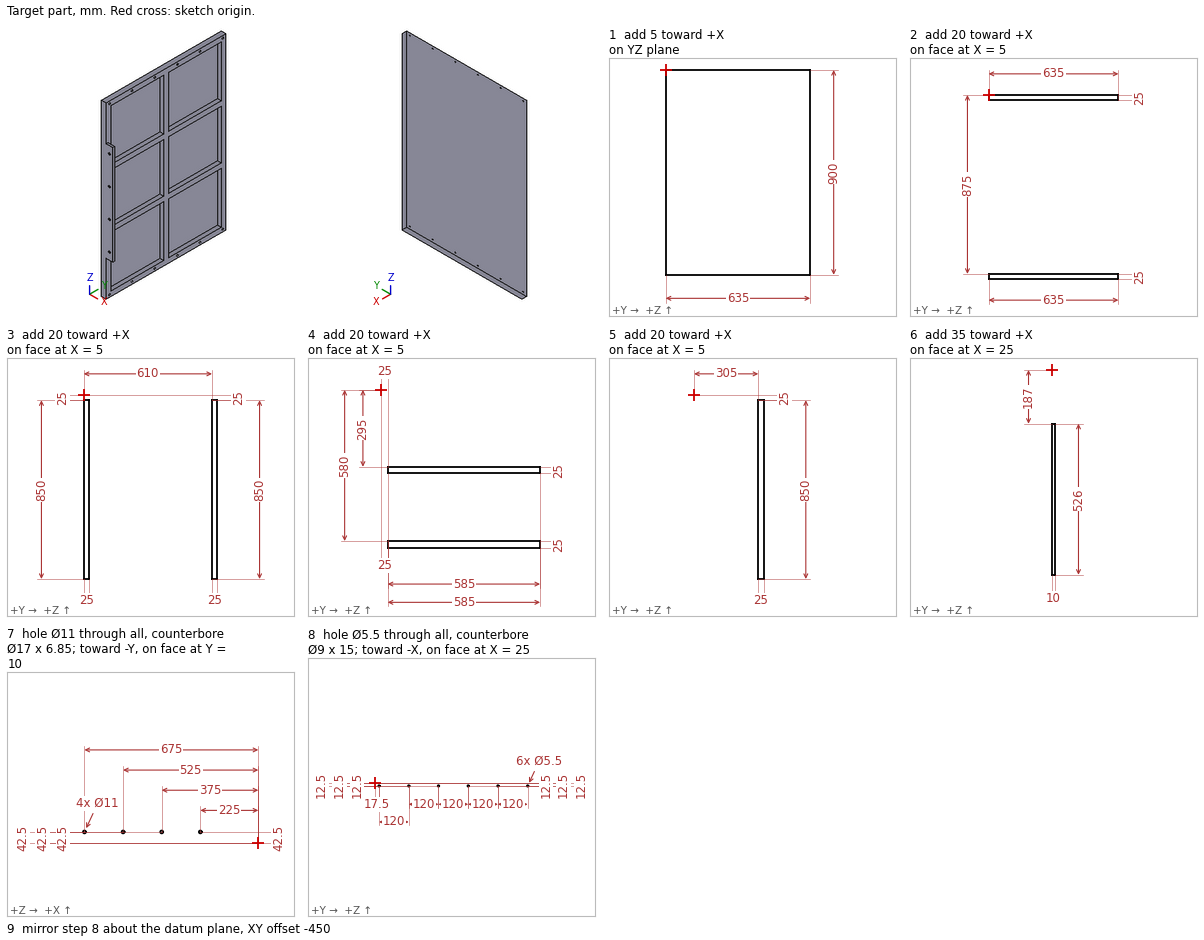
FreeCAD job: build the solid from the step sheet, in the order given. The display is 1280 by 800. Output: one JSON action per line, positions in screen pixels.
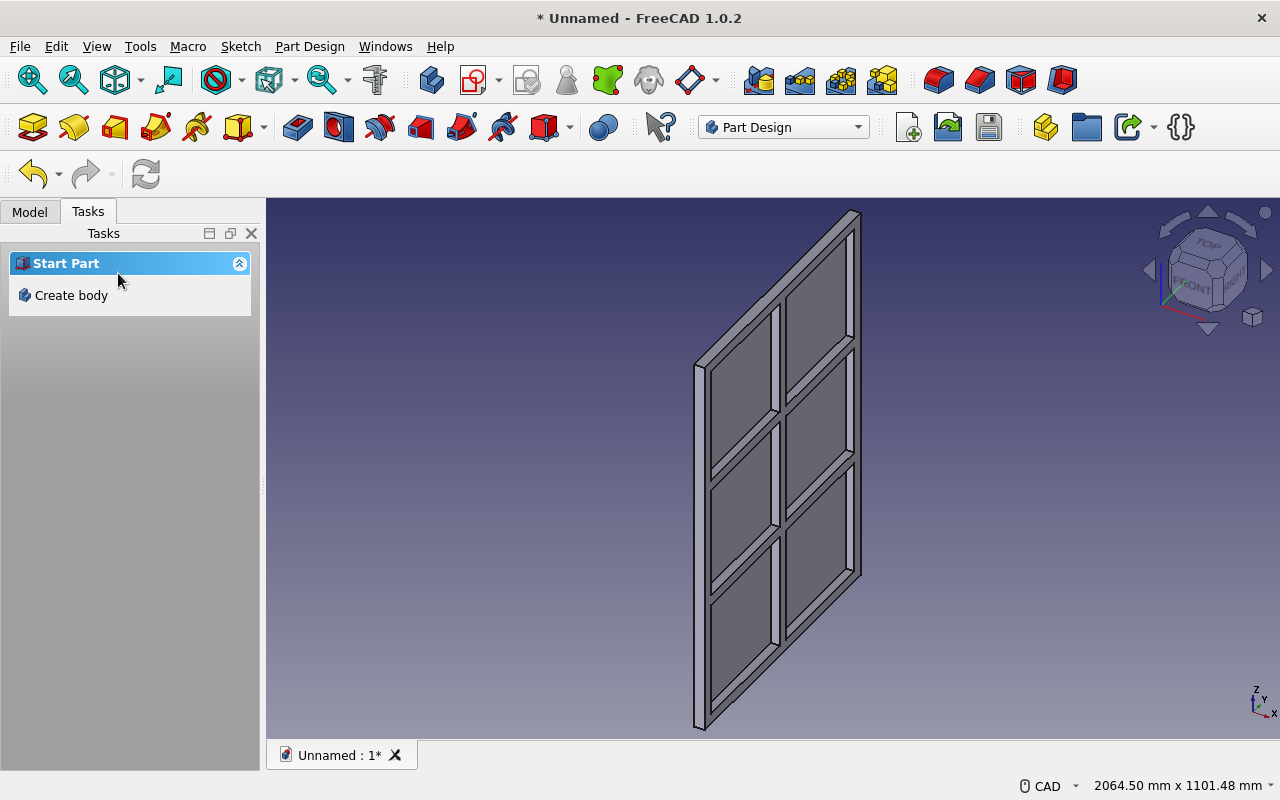
{"action": "scroll", "coordinate": [783, 626], "scroll_direction": "up", "scroll_amount": 4}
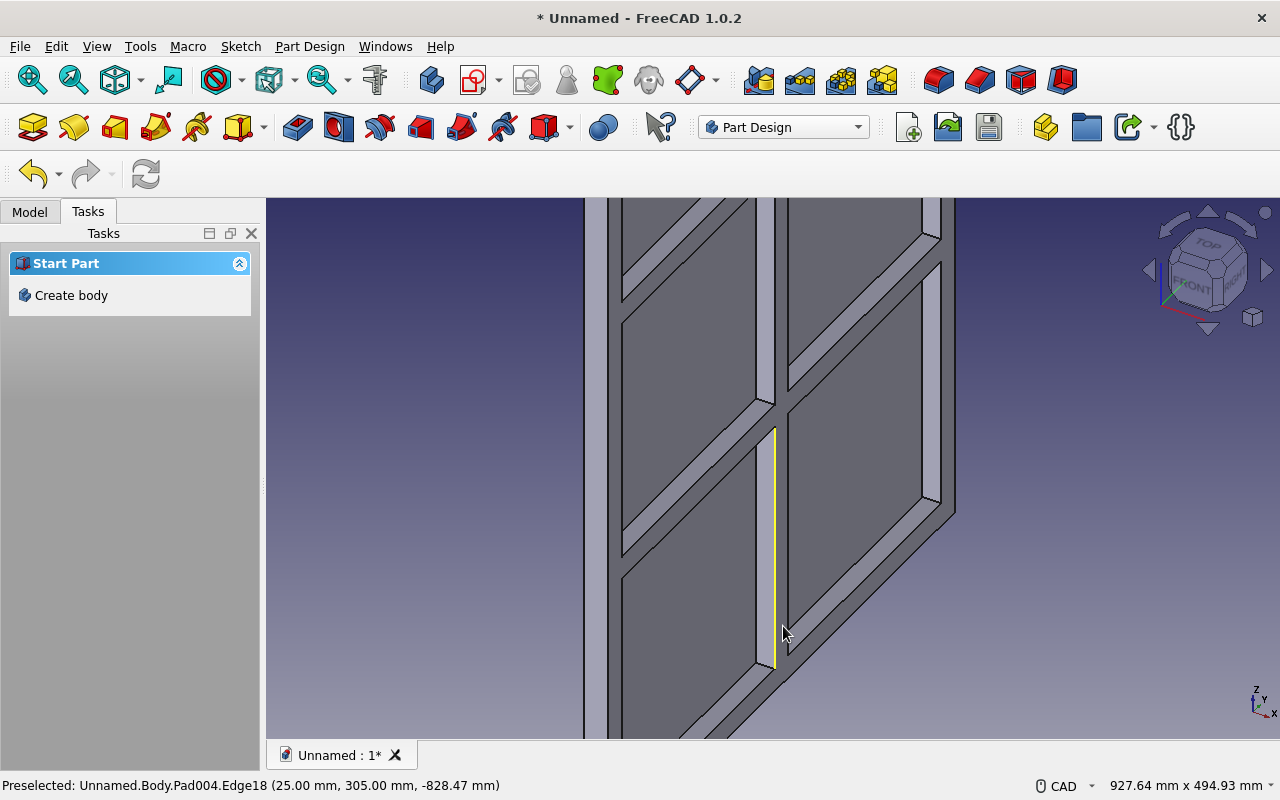
{"action": "left_click", "coordinate": [33, 80]}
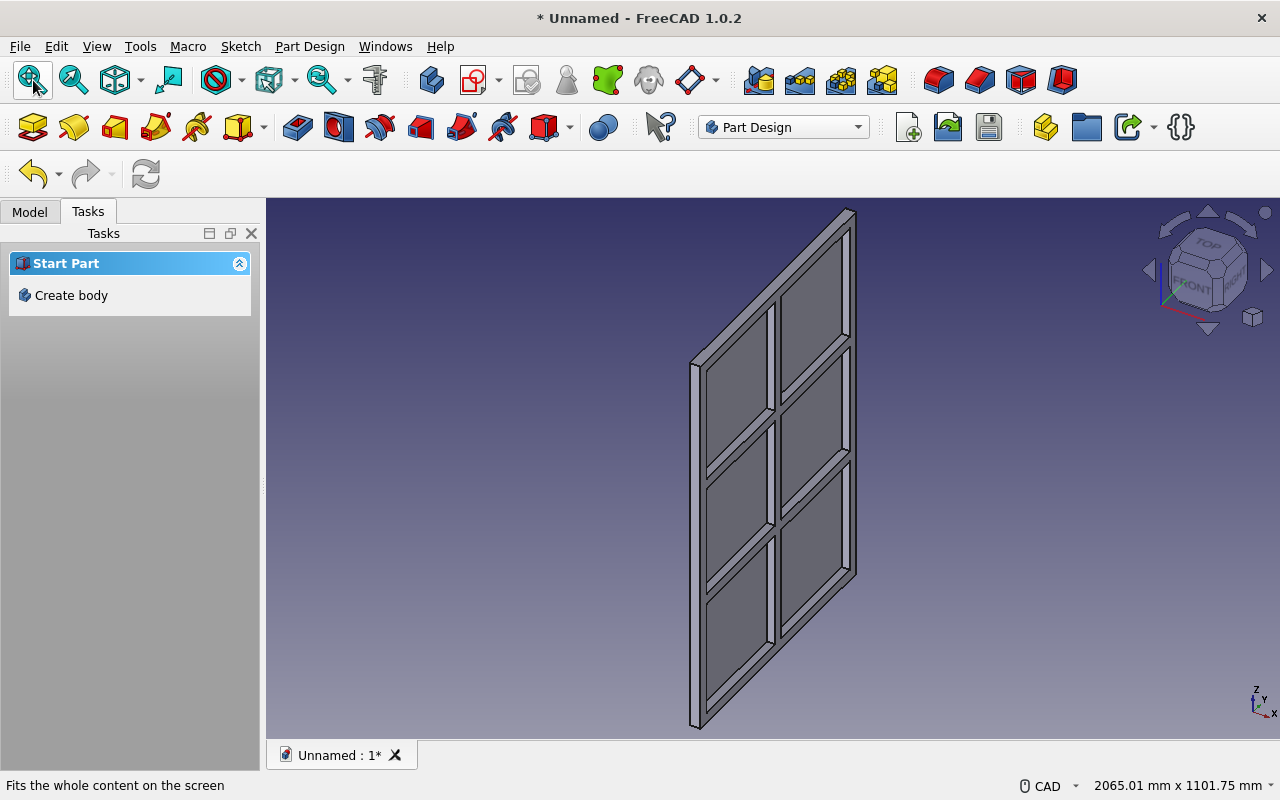
{"action": "key", "text": "0"}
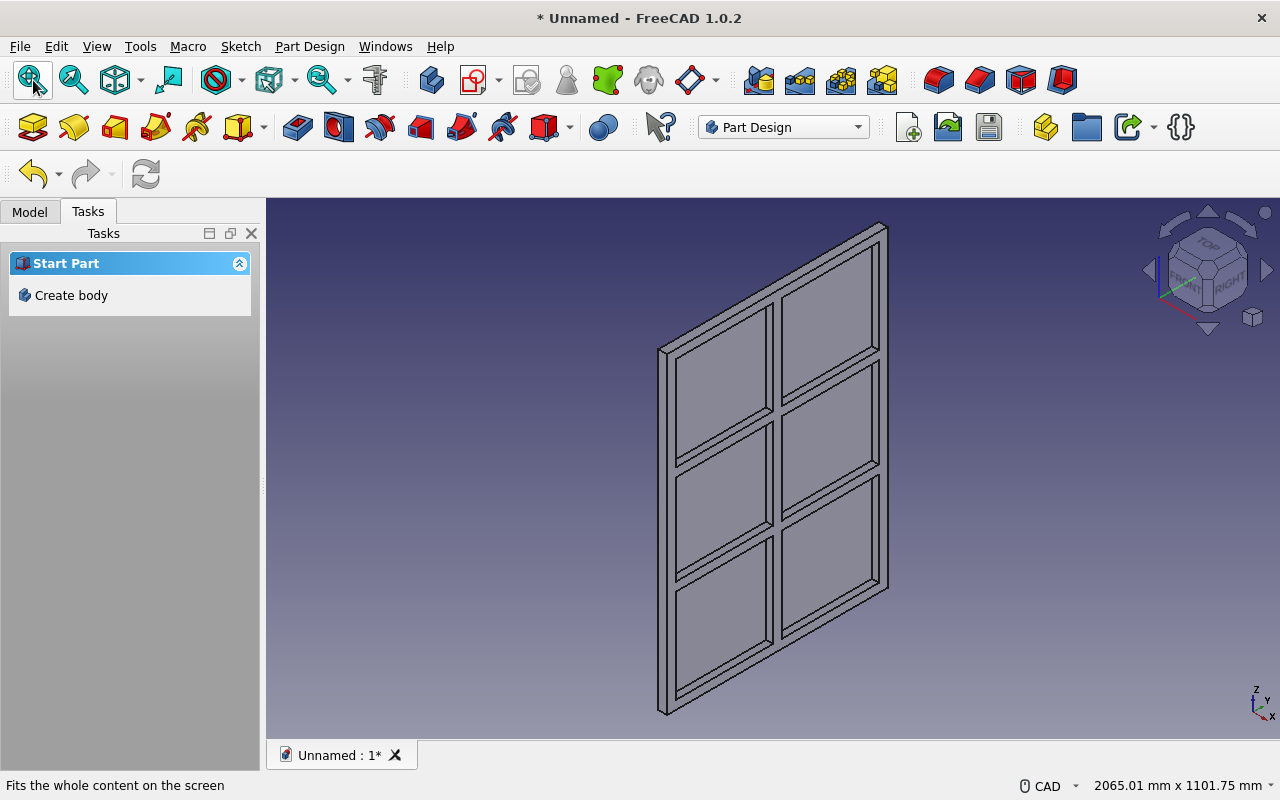
{"action": "scroll", "coordinate": [777, 625], "scroll_direction": "up", "scroll_amount": 4}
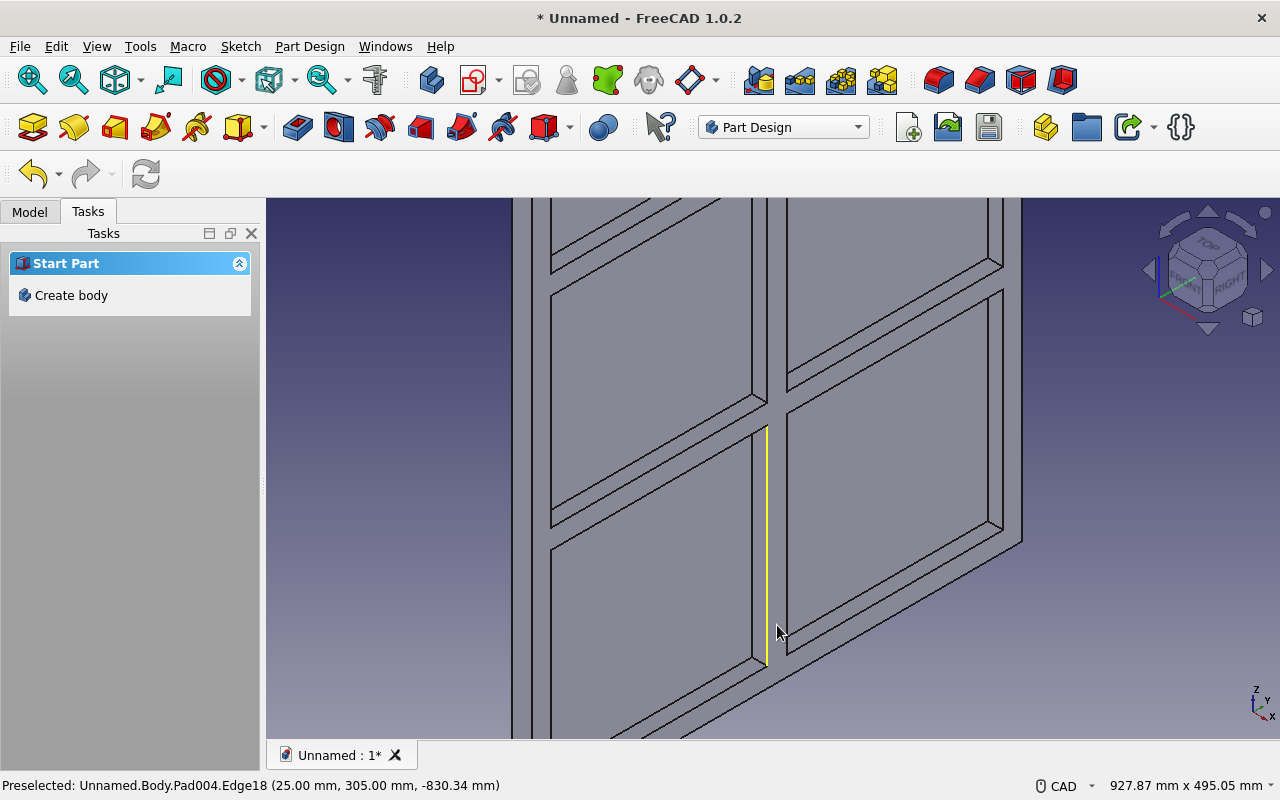
{"action": "left_click", "coordinate": [777, 624]}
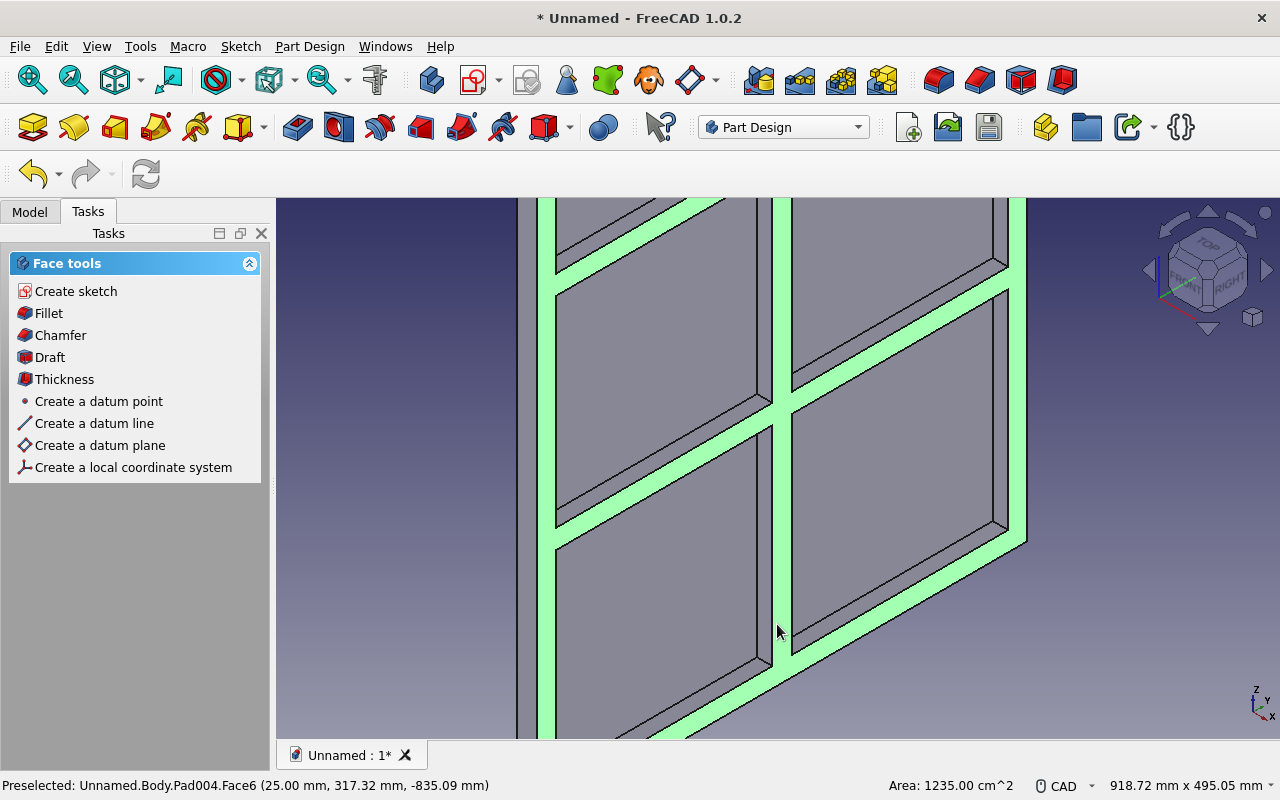
{"action": "left_click", "coordinate": [472, 80]}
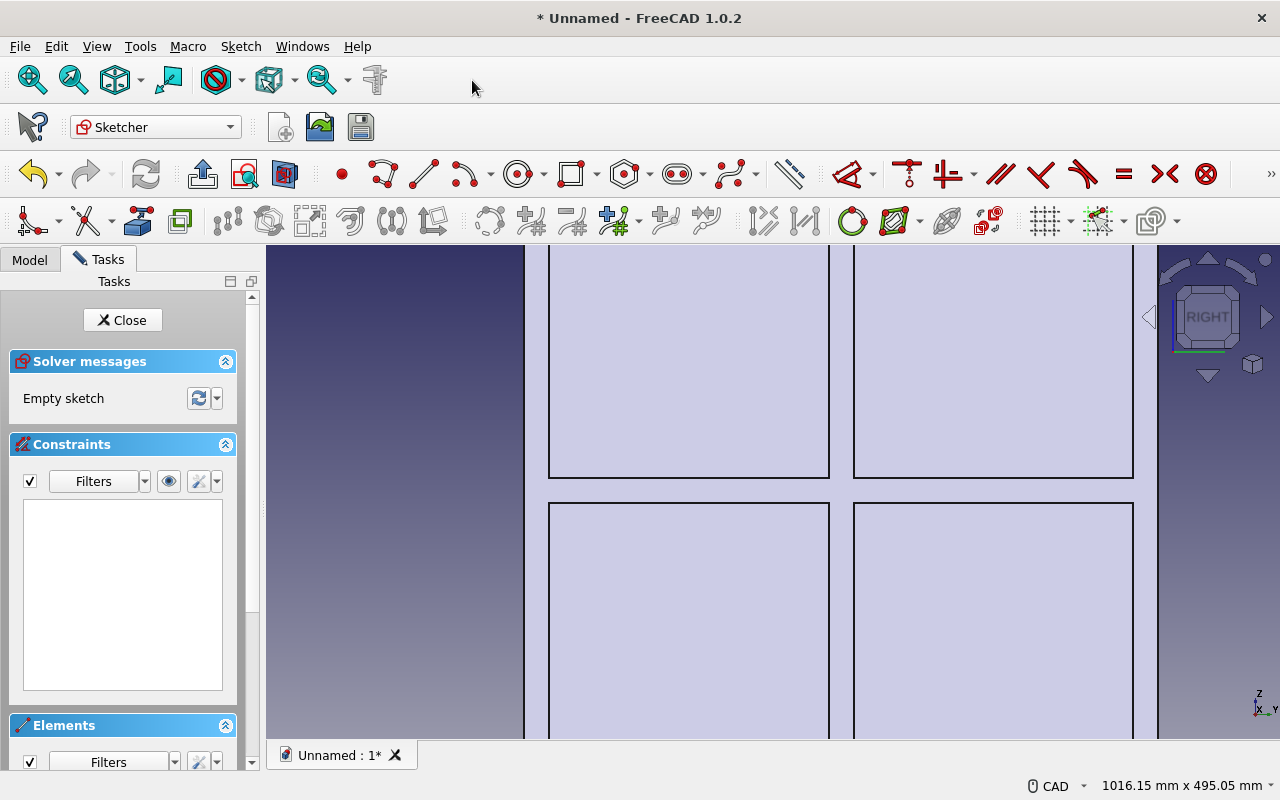
{"action": "scroll", "coordinate": [847, 685], "scroll_direction": "down", "scroll_amount": 4}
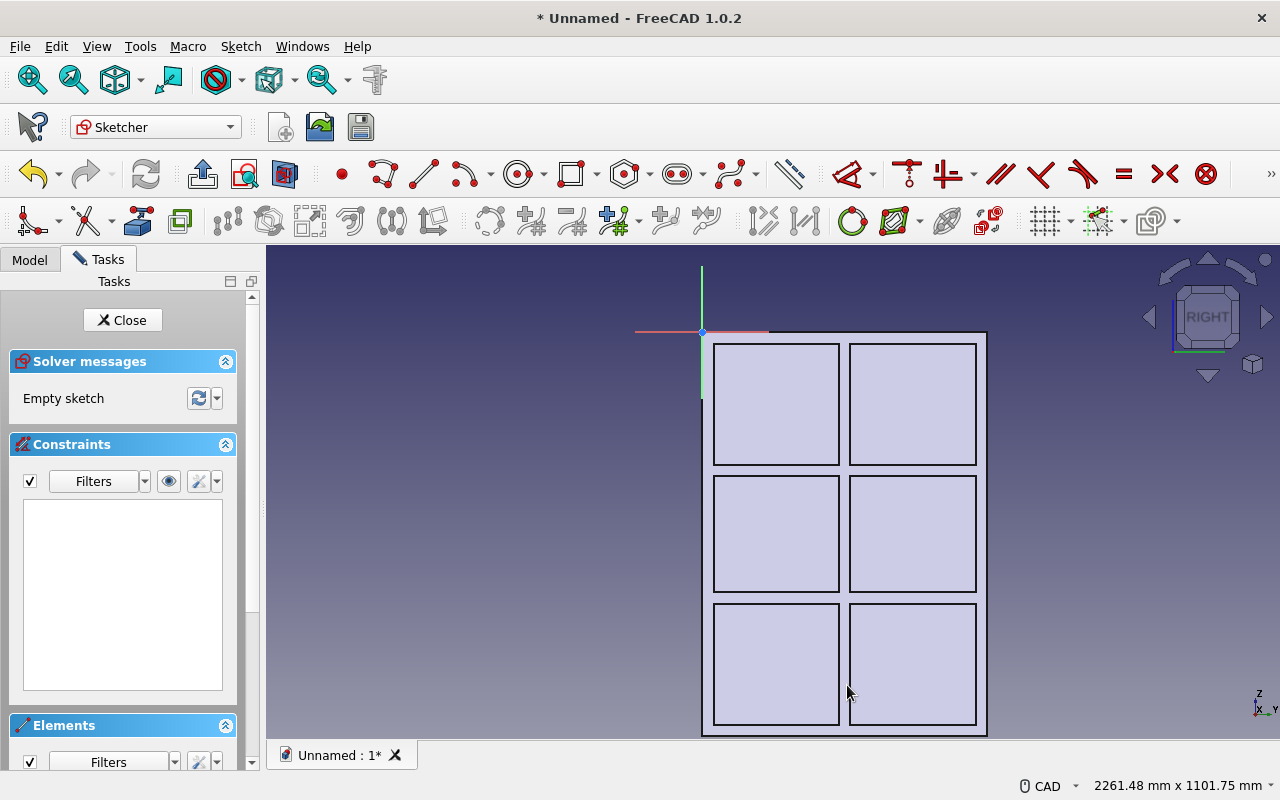
{"action": "left_click", "coordinate": [570, 174]}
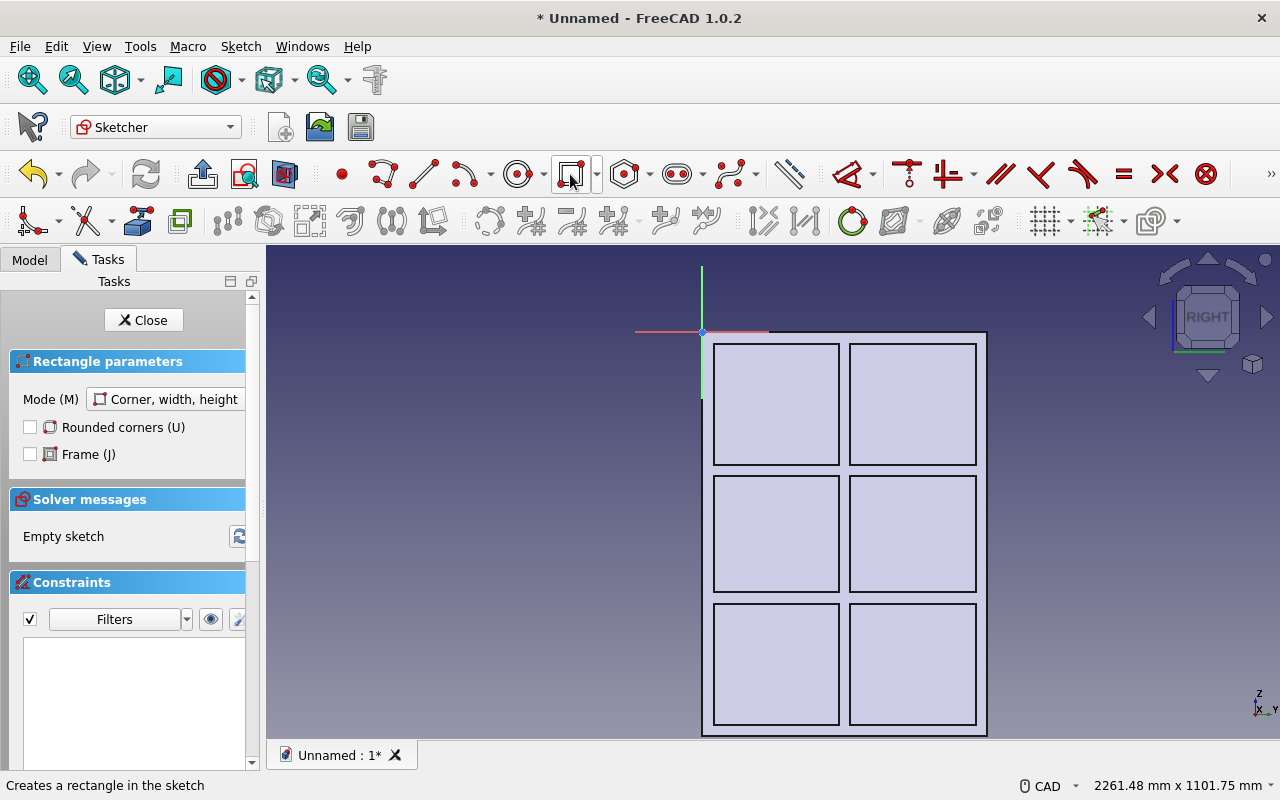
{"action": "scroll", "coordinate": [702, 416], "scroll_direction": "up", "scroll_amount": 7}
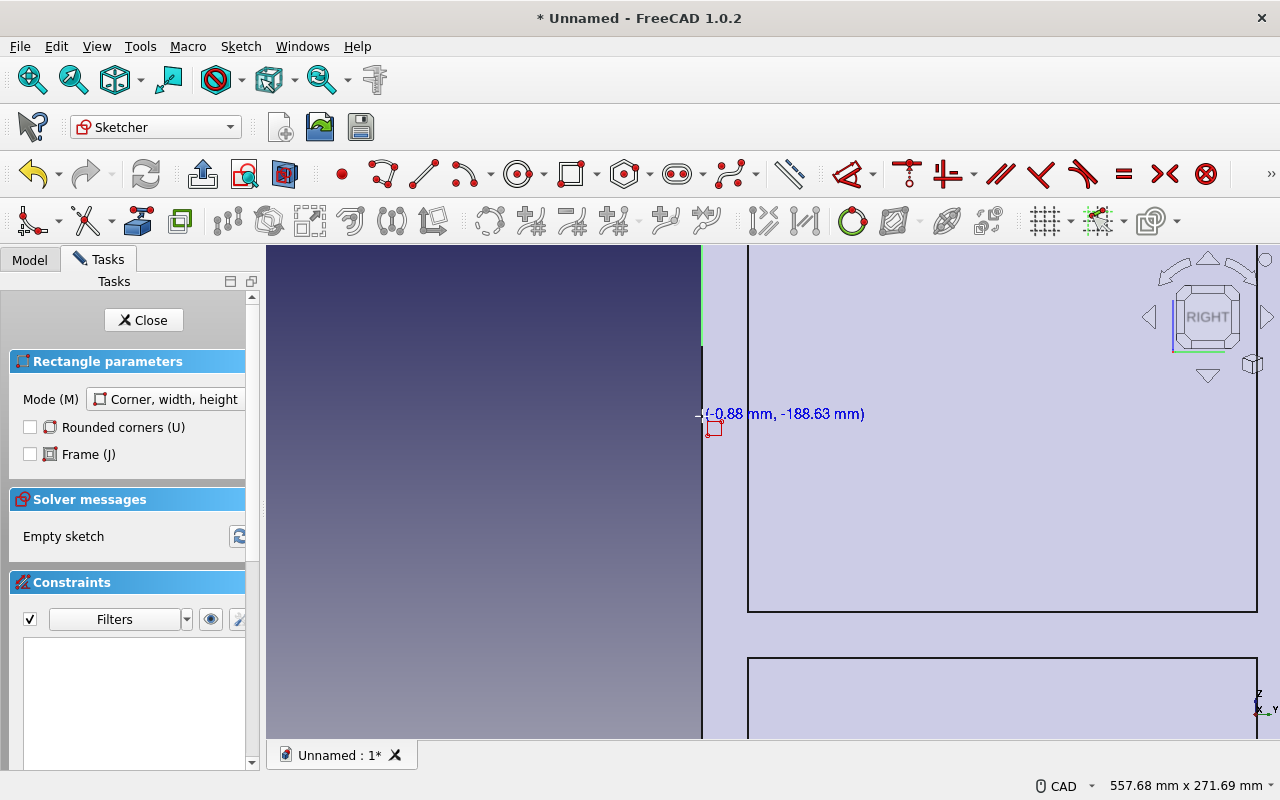
{"action": "scroll", "coordinate": [702, 416], "scroll_direction": "down", "scroll_amount": 7}